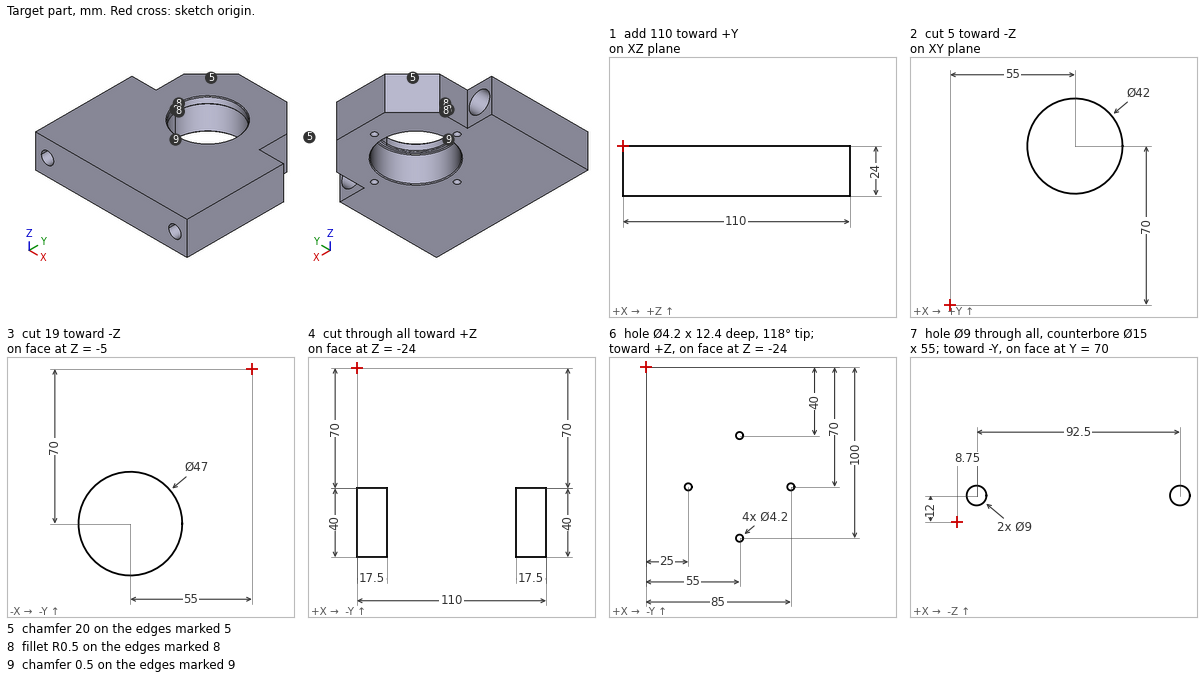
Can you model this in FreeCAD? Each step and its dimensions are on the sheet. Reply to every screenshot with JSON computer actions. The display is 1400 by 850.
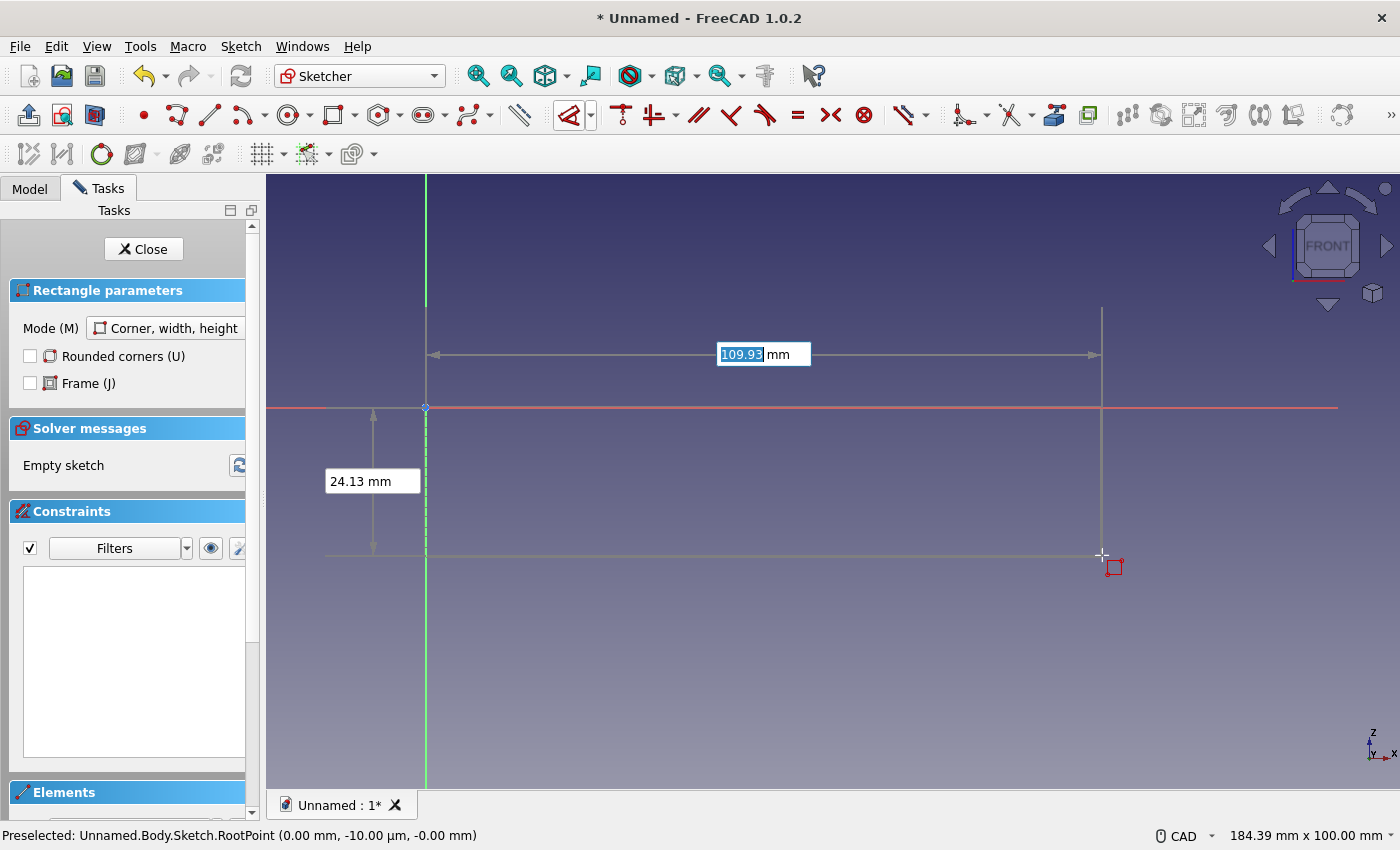
{"action": "type", "text": "110"}
{"action": "key", "text": "Tab"}
{"action": "type", "text": "24"}
{"action": "key", "text": "Return"}
{"action": "key", "text": "Escape"}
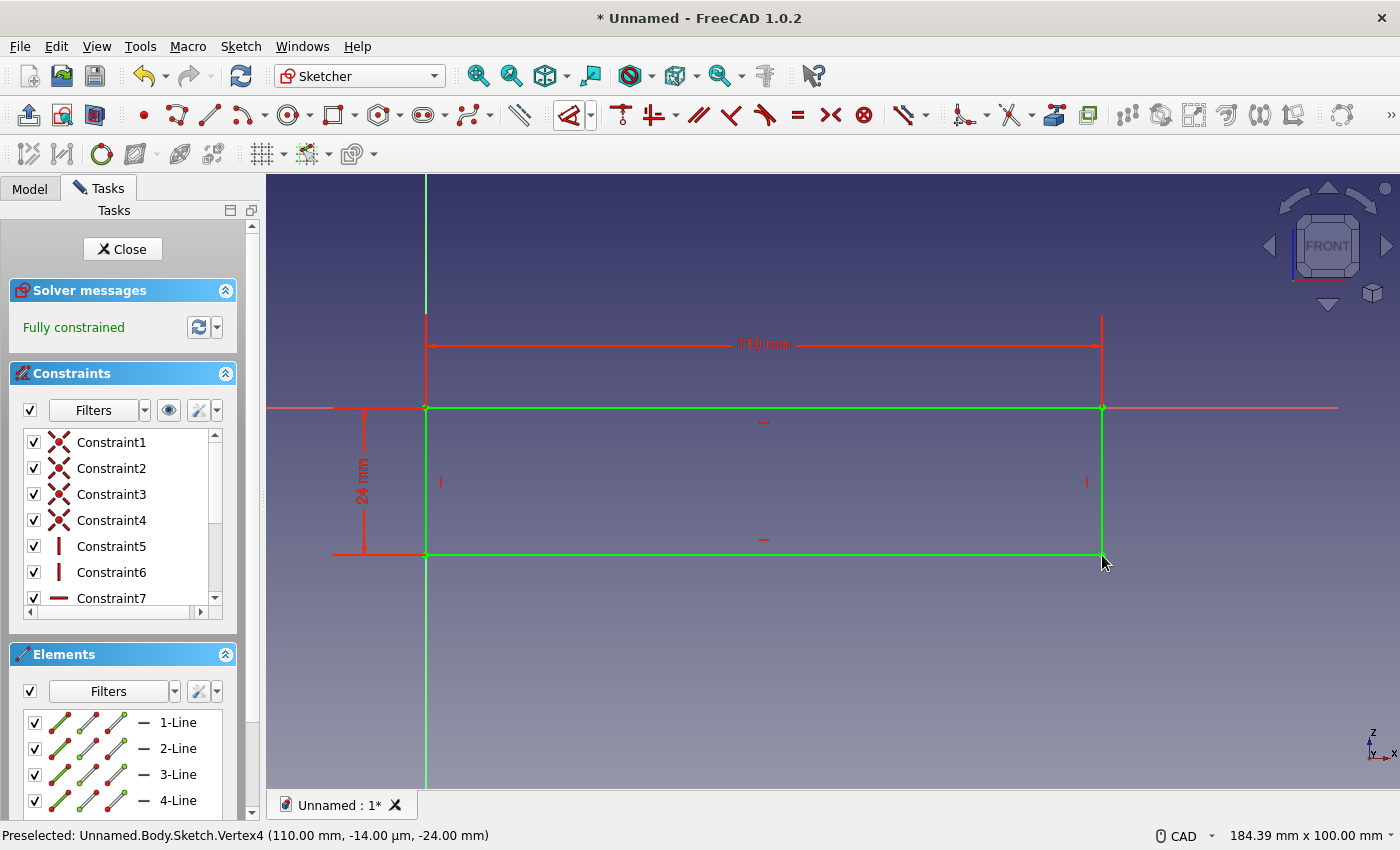
{"action": "left_click", "coordinate": [123, 249]}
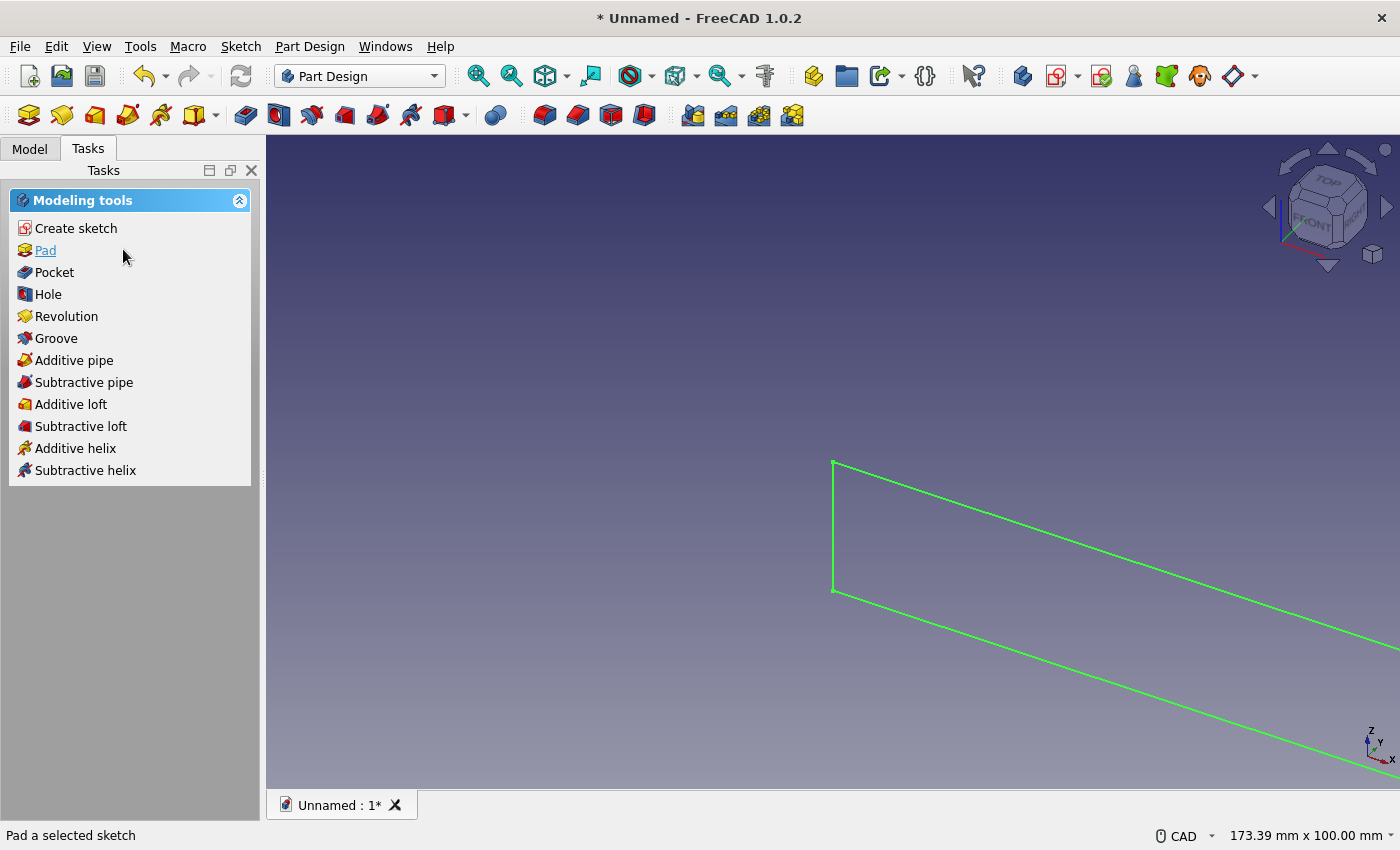
{"action": "left_click", "coordinate": [29, 116]}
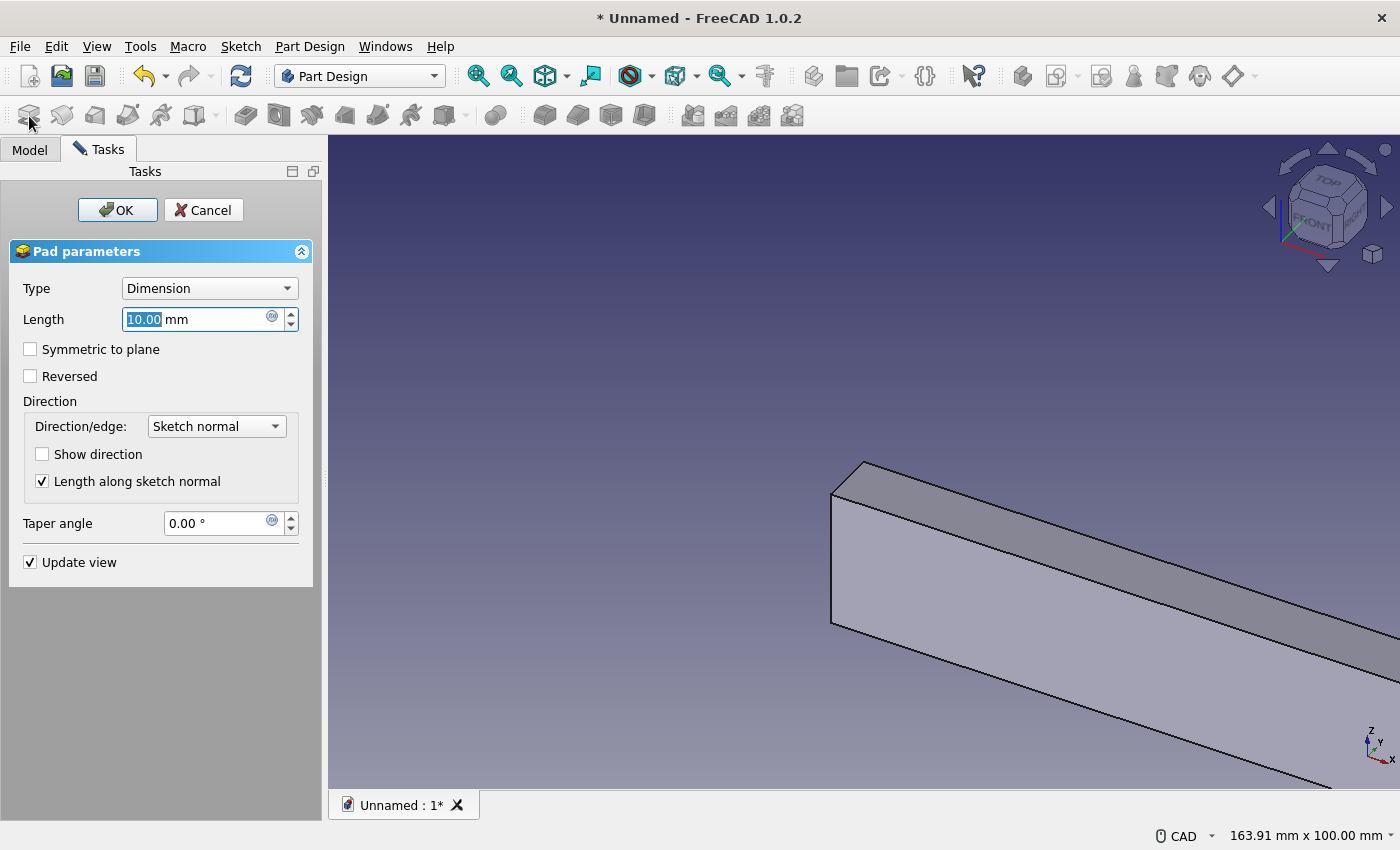
{"action": "type", "text": "110"}
{"action": "key", "text": "Tab"}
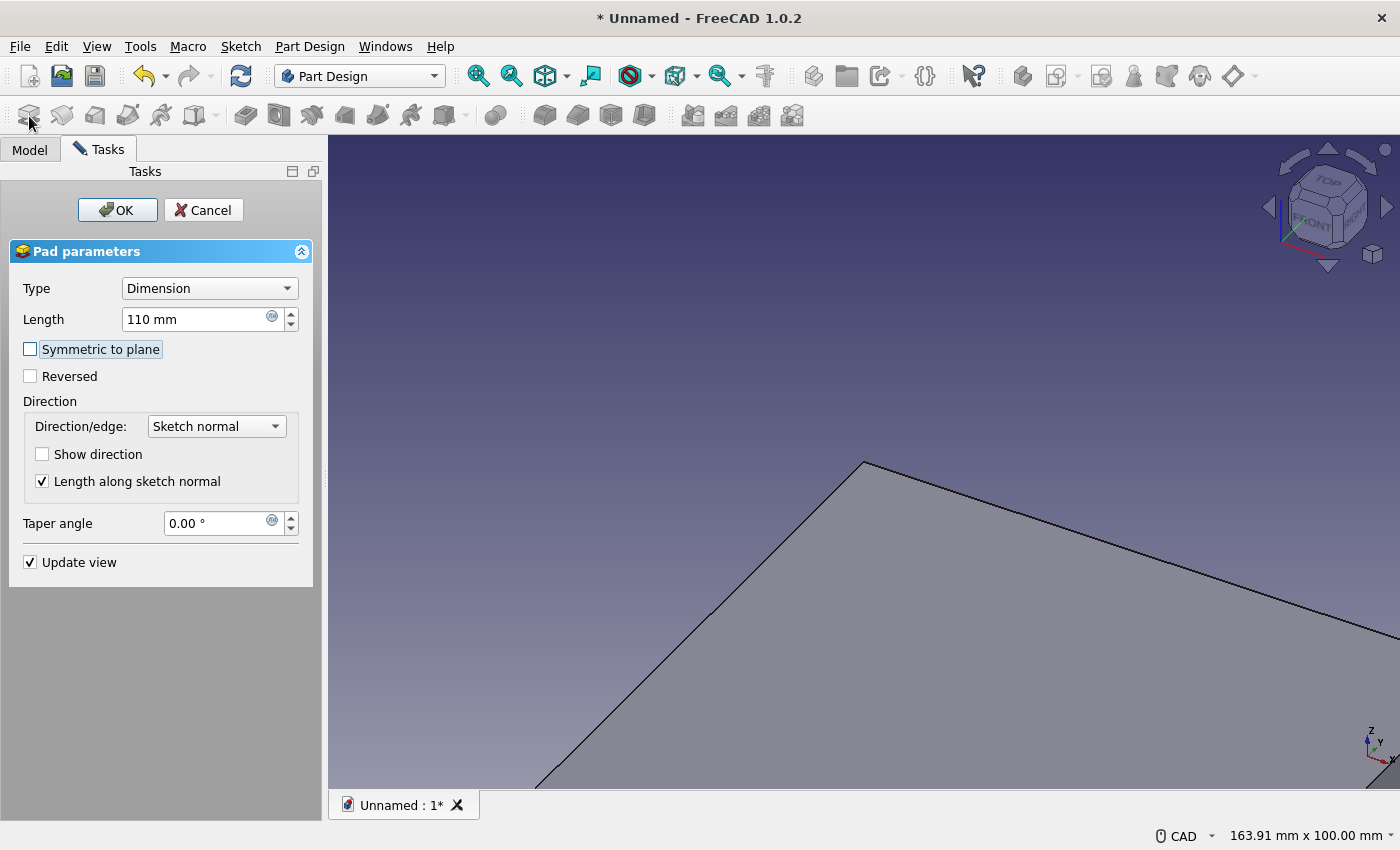
{"action": "left_click", "coordinate": [31, 376]}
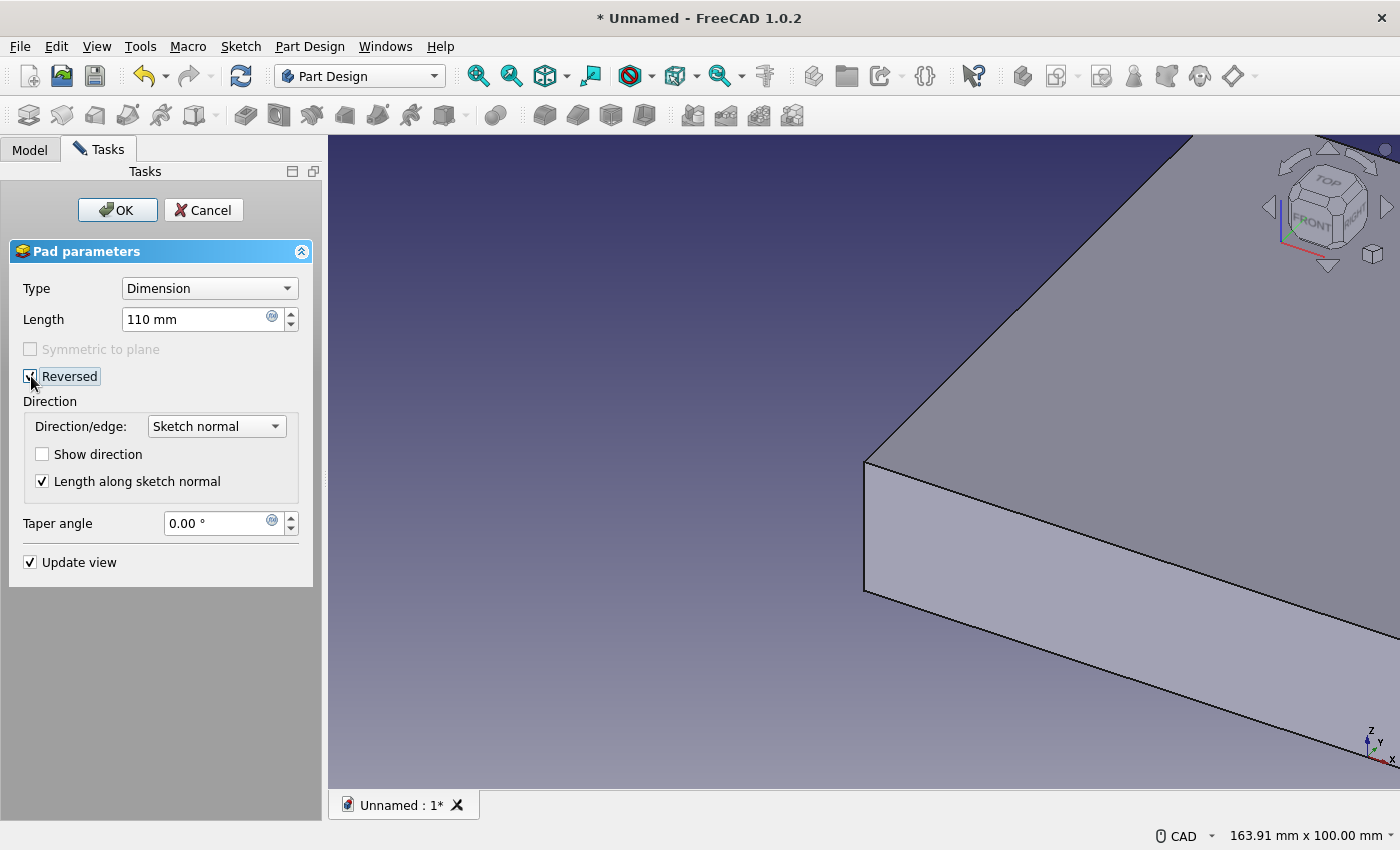
{"action": "left_click", "coordinate": [118, 210]}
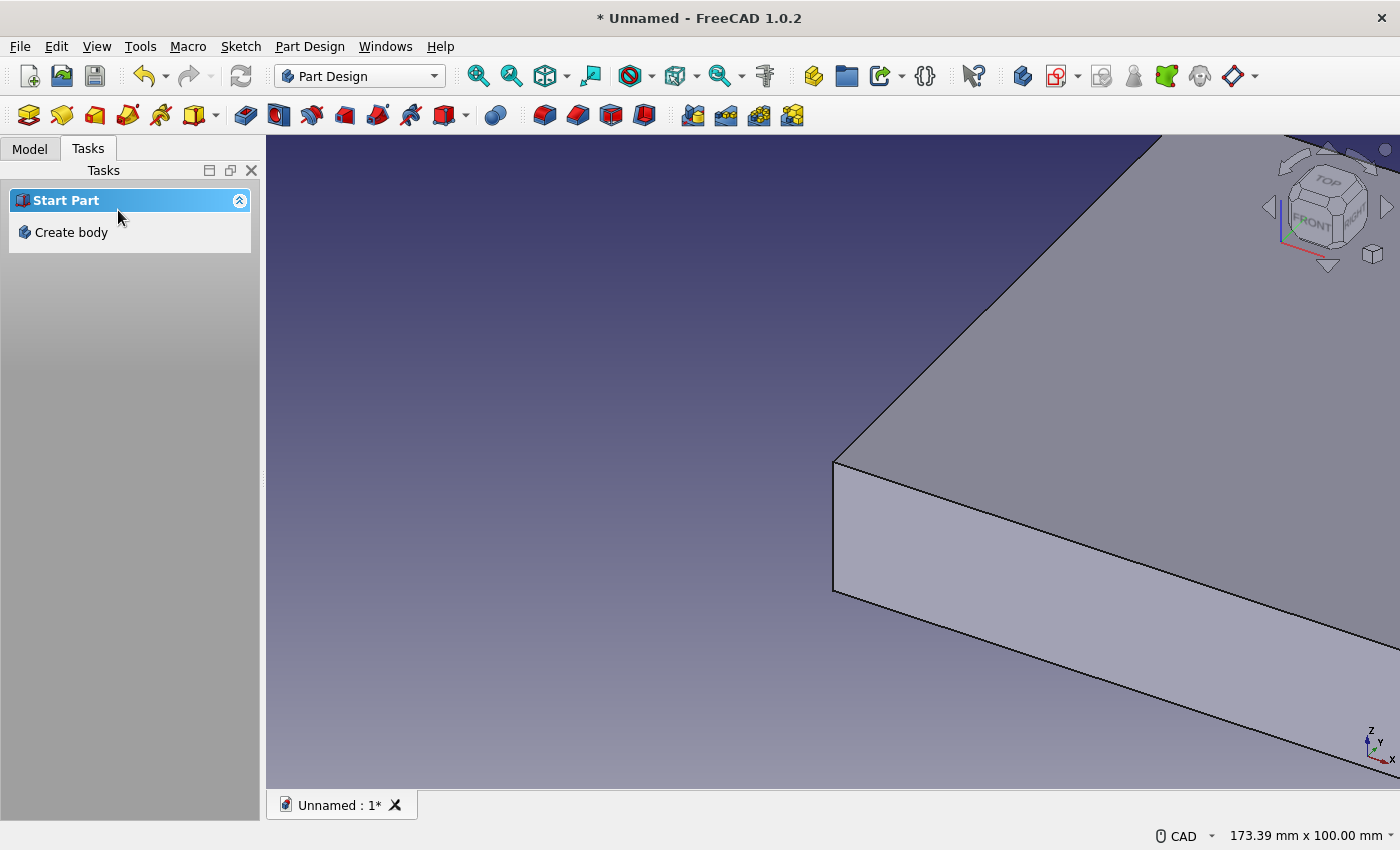
{"action": "key", "text": "v f"}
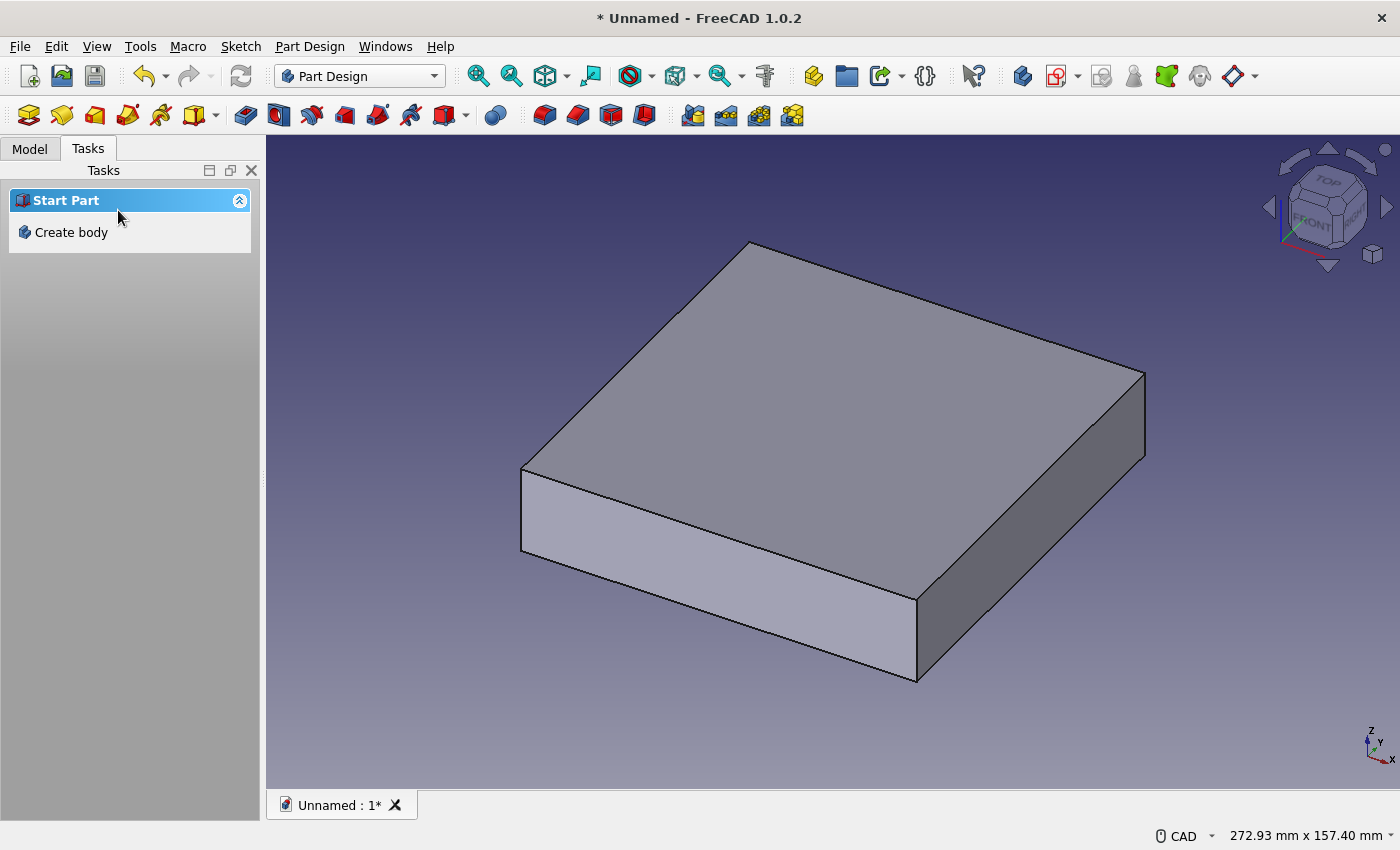
{"action": "left_click", "coordinate": [1056, 76]}